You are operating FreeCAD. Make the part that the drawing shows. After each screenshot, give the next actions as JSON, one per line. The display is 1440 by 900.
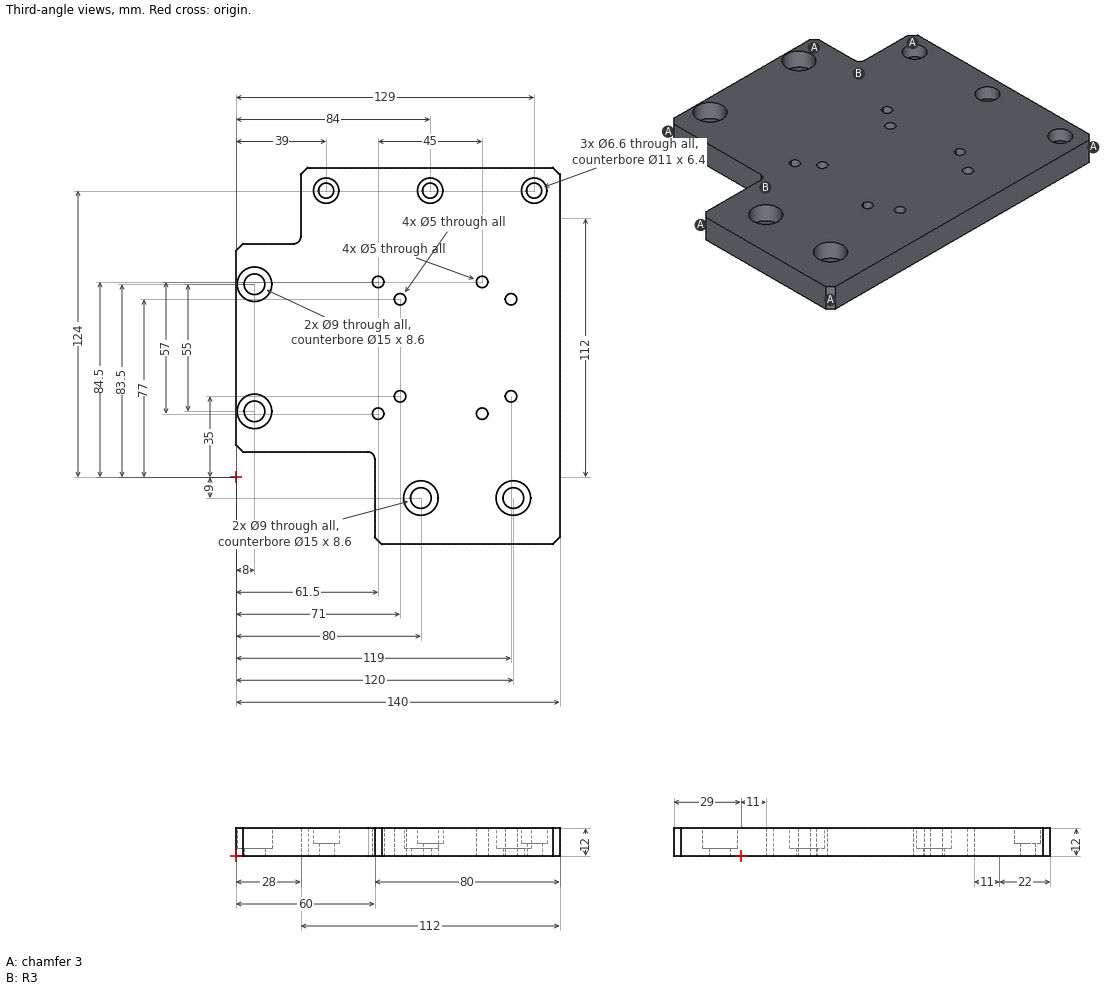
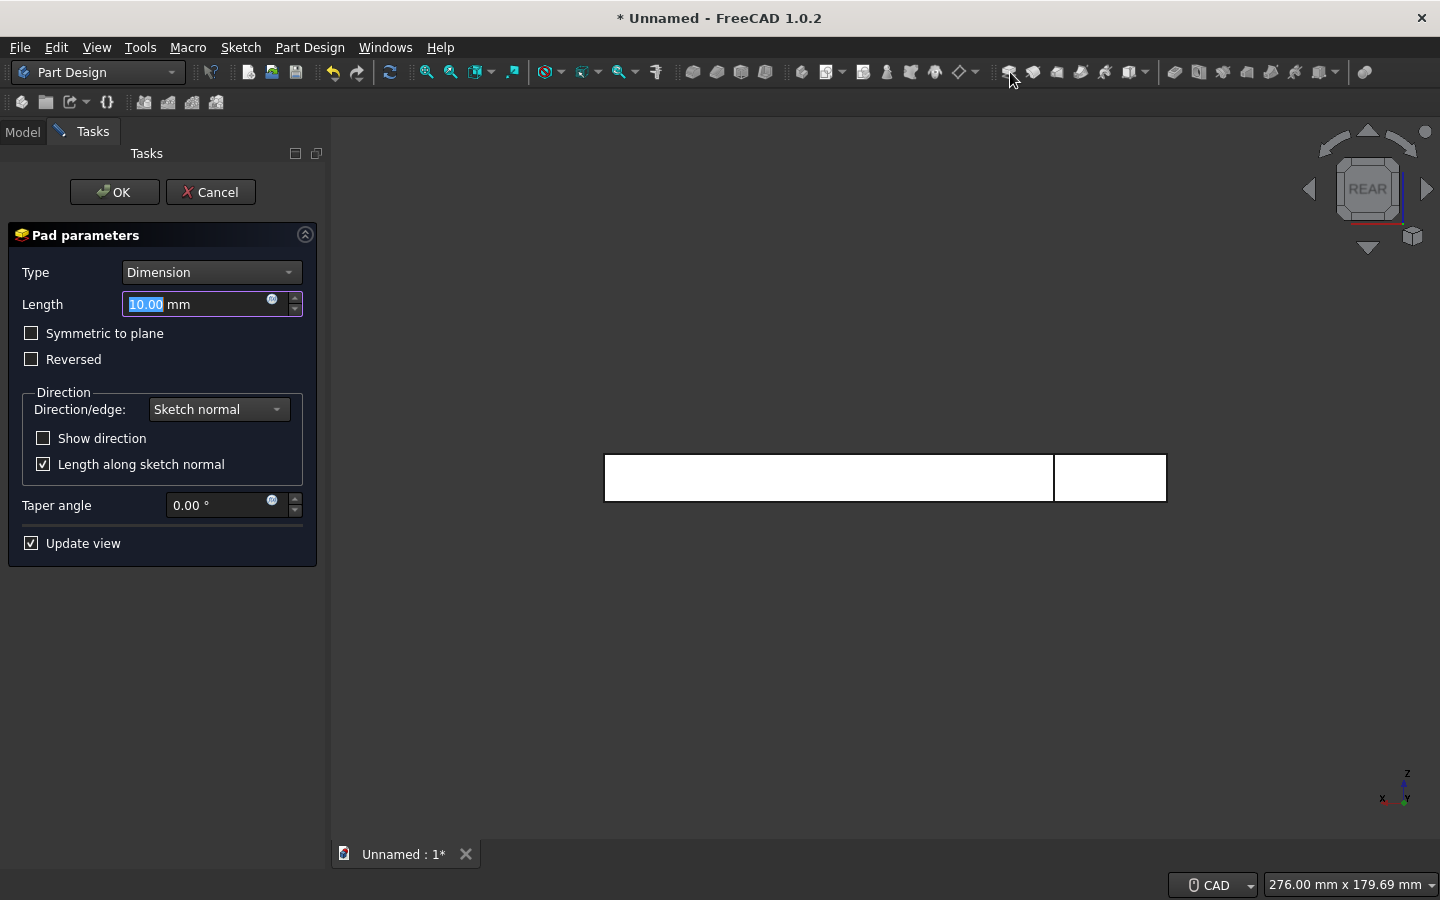
{"action": "type", "text": "22"}
{"action": "key", "text": "Tab"}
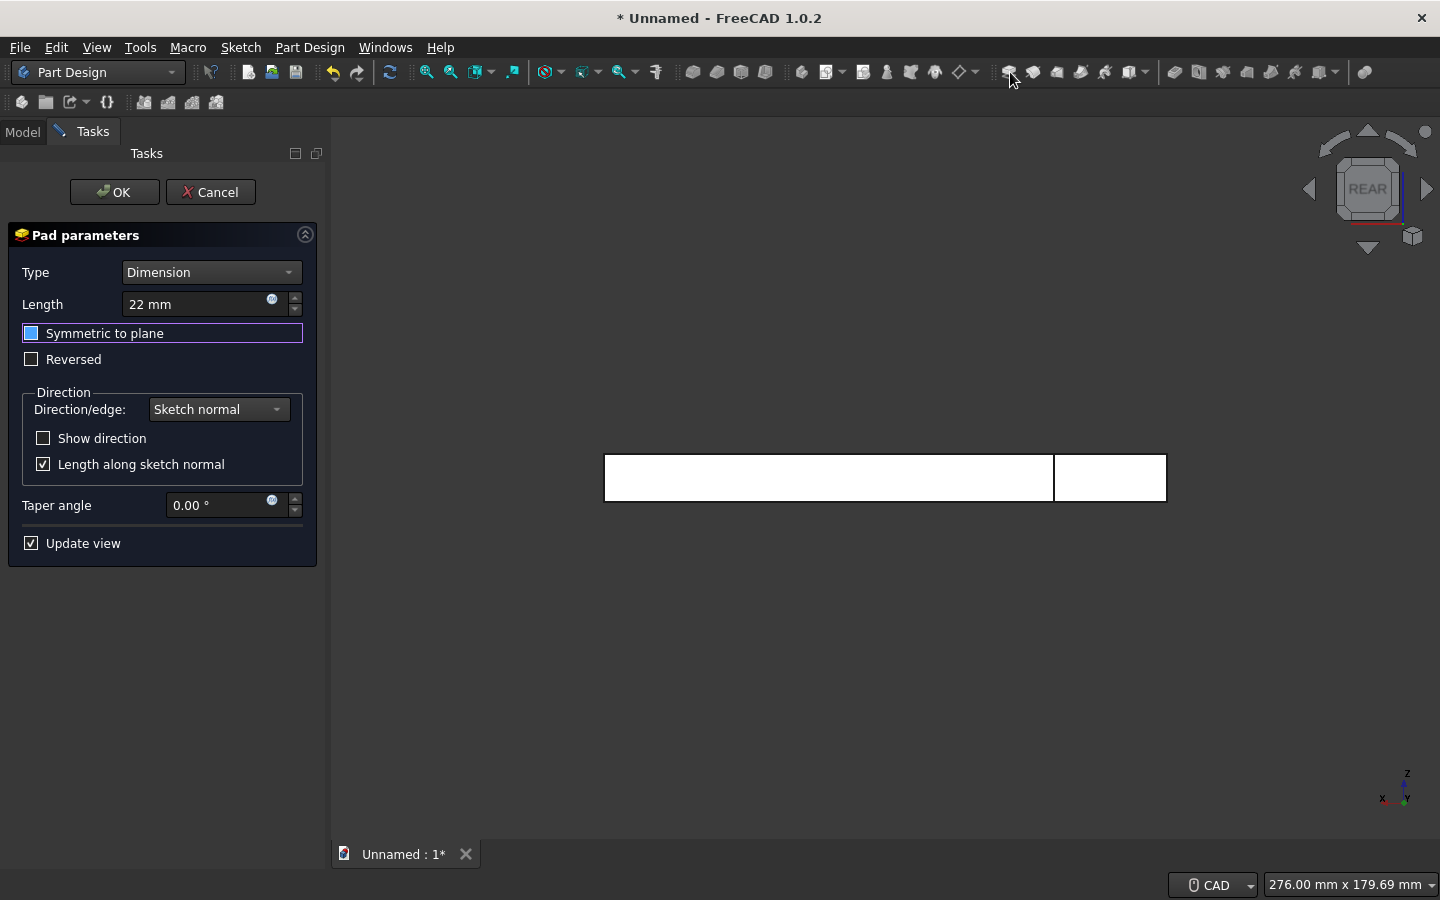
{"action": "left_click", "coordinate": [115, 192]}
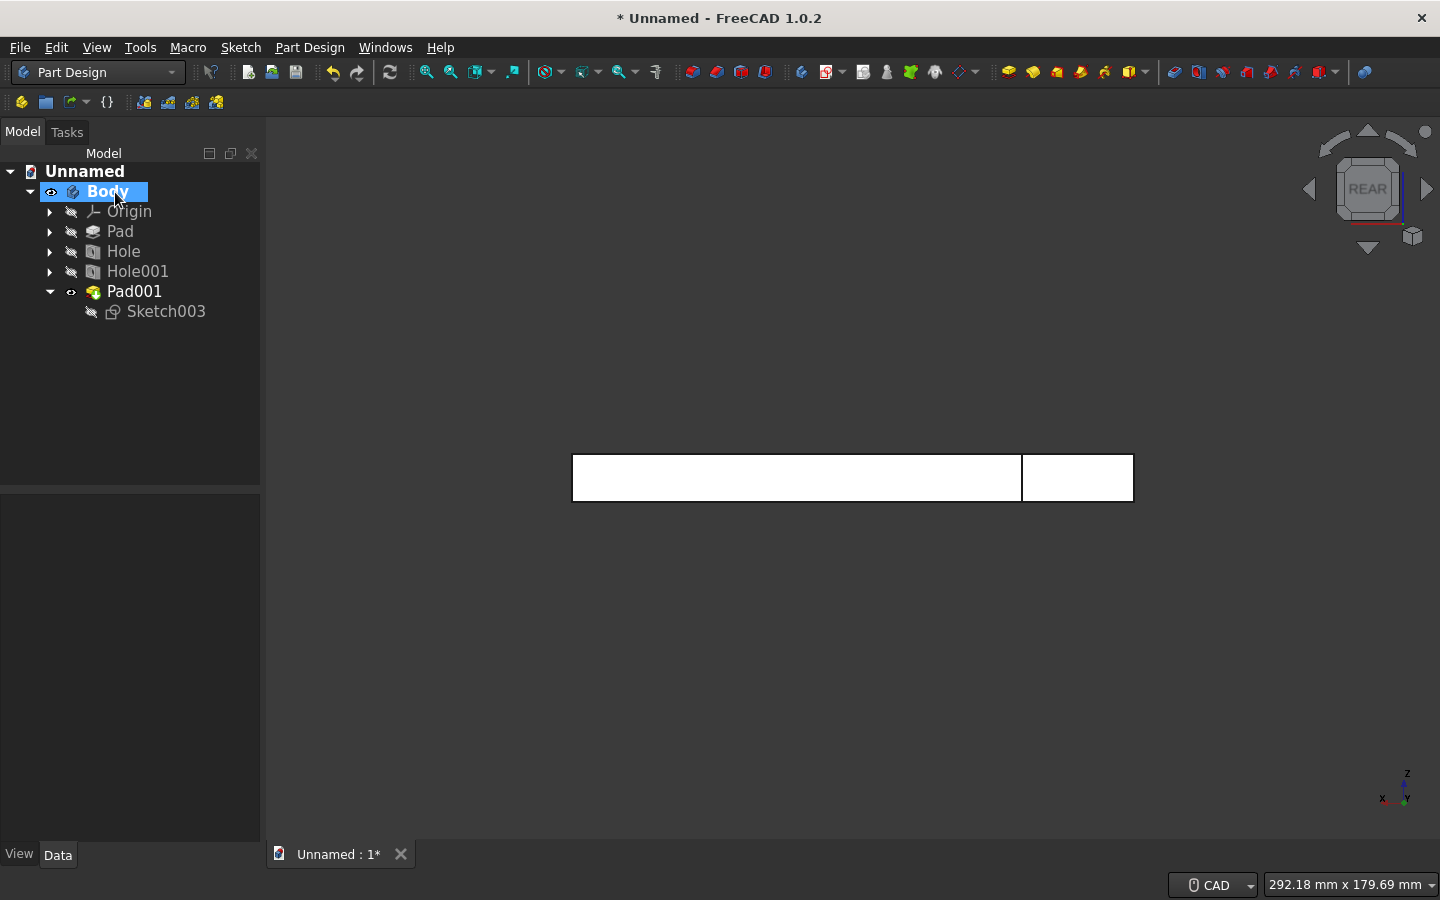
{"action": "left_click", "coordinate": [1046, 477]}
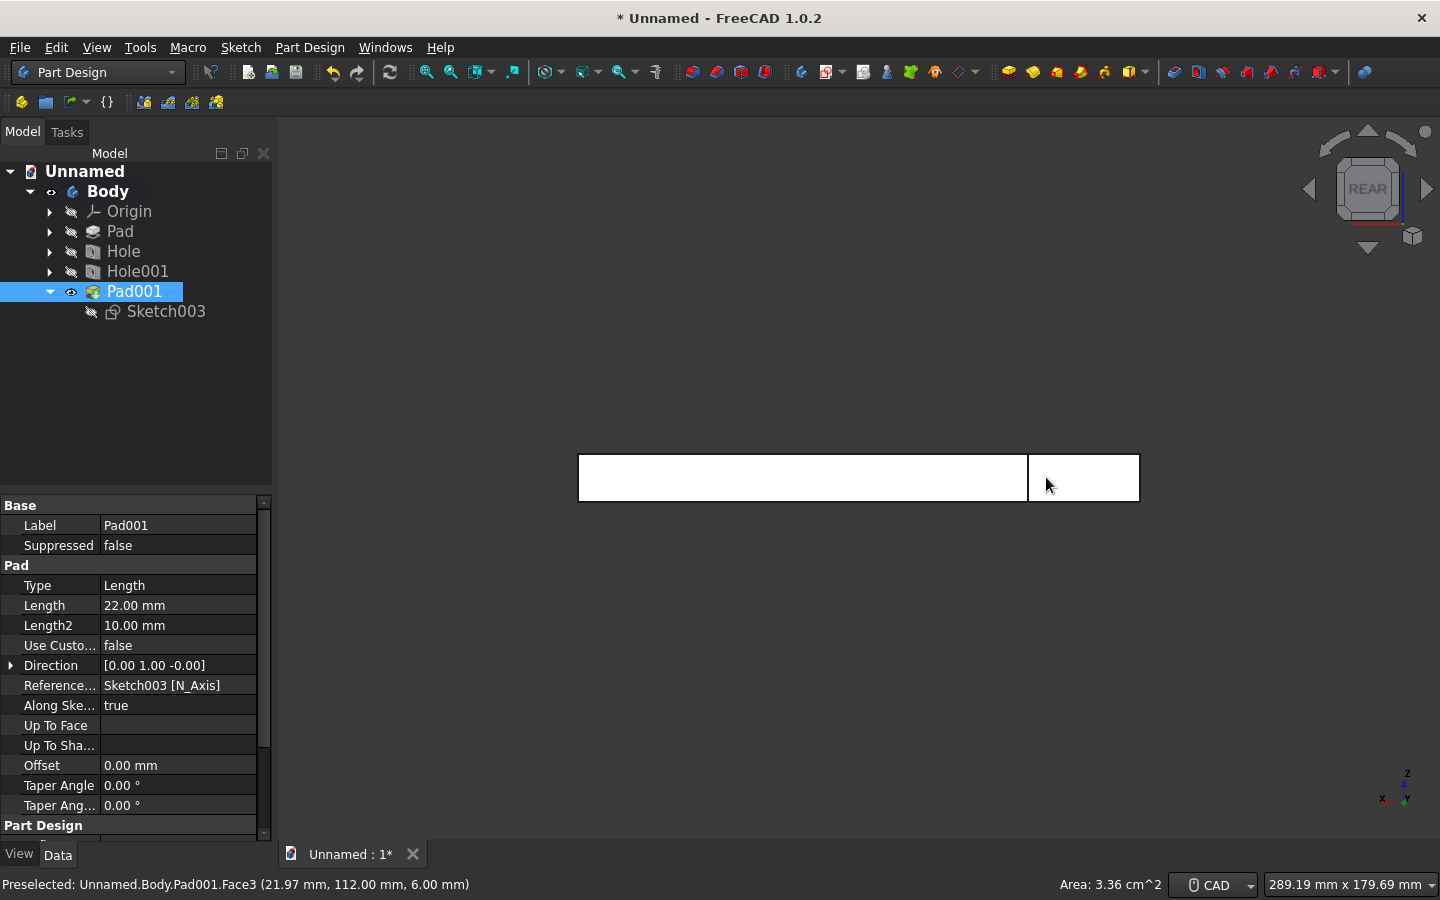
{"action": "left_click", "coordinate": [826, 72]}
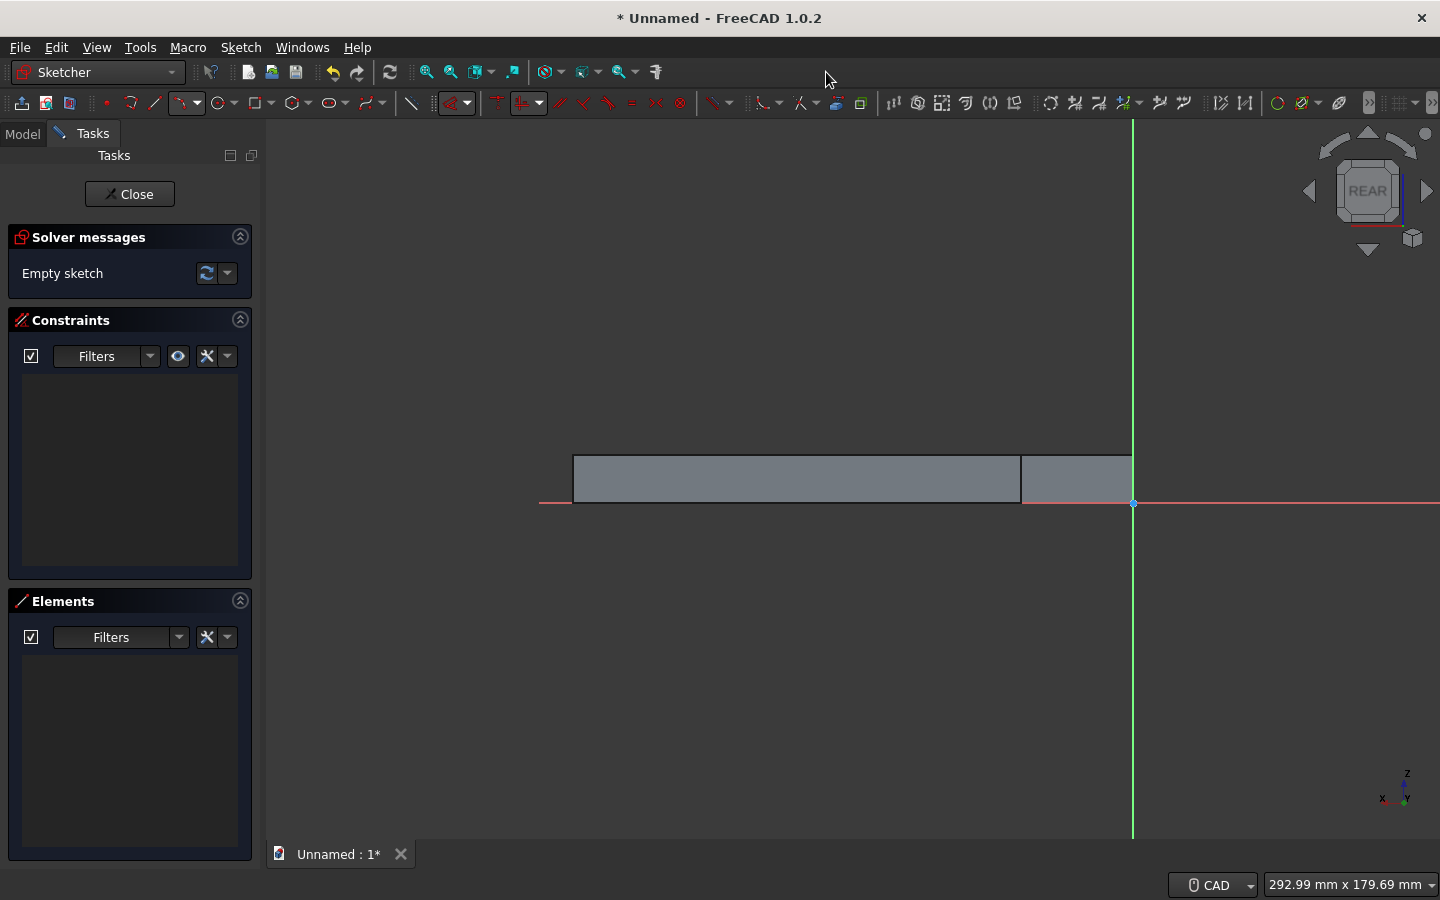
{"action": "left_click", "coordinate": [70, 104]}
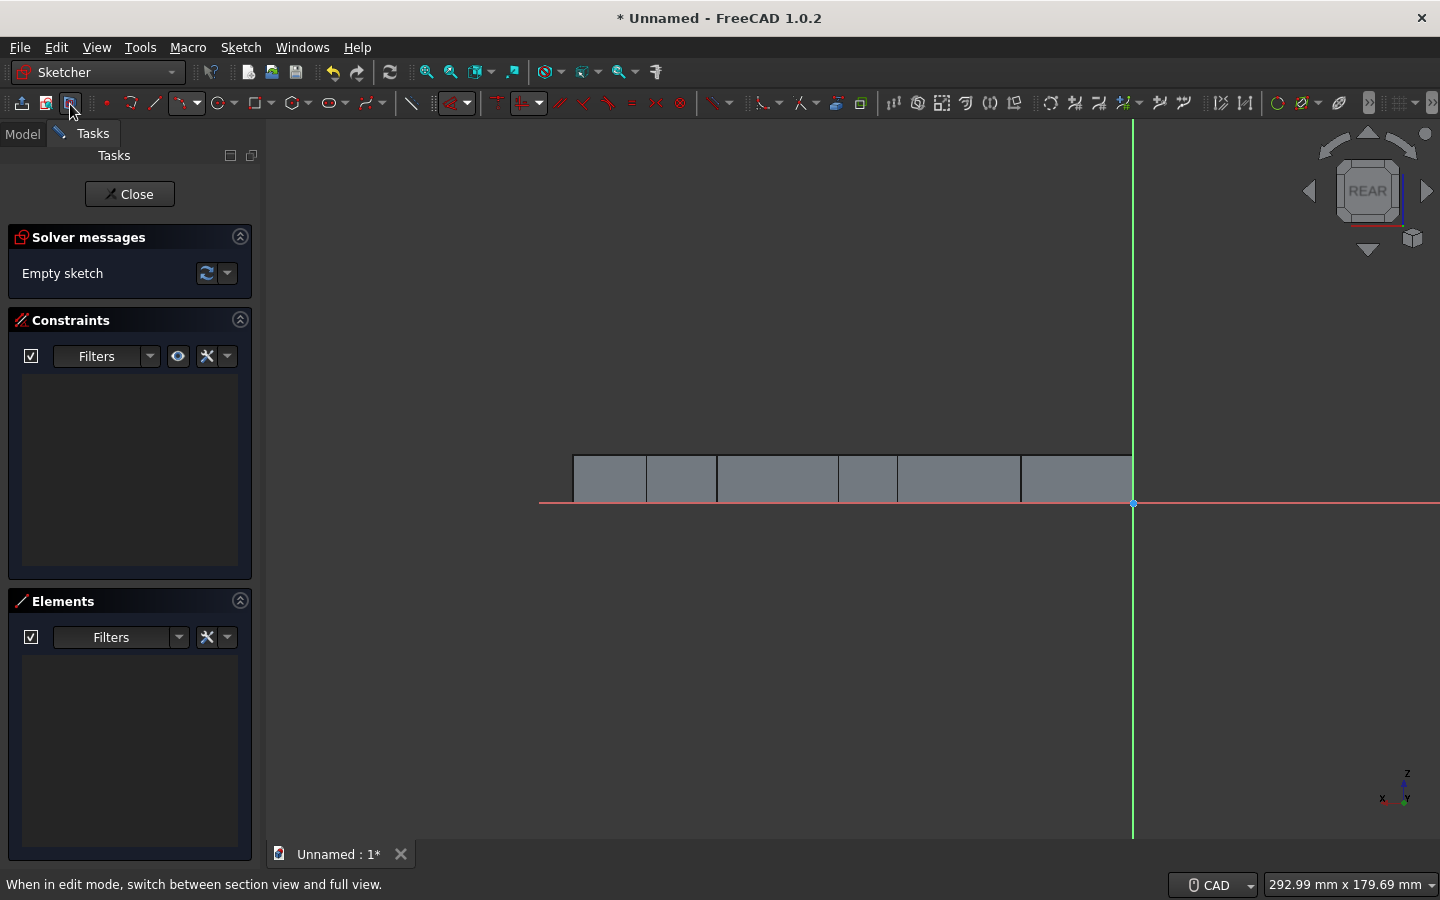
{"action": "scroll", "coordinate": [1135, 479], "scroll_direction": "up", "scroll_amount": 9}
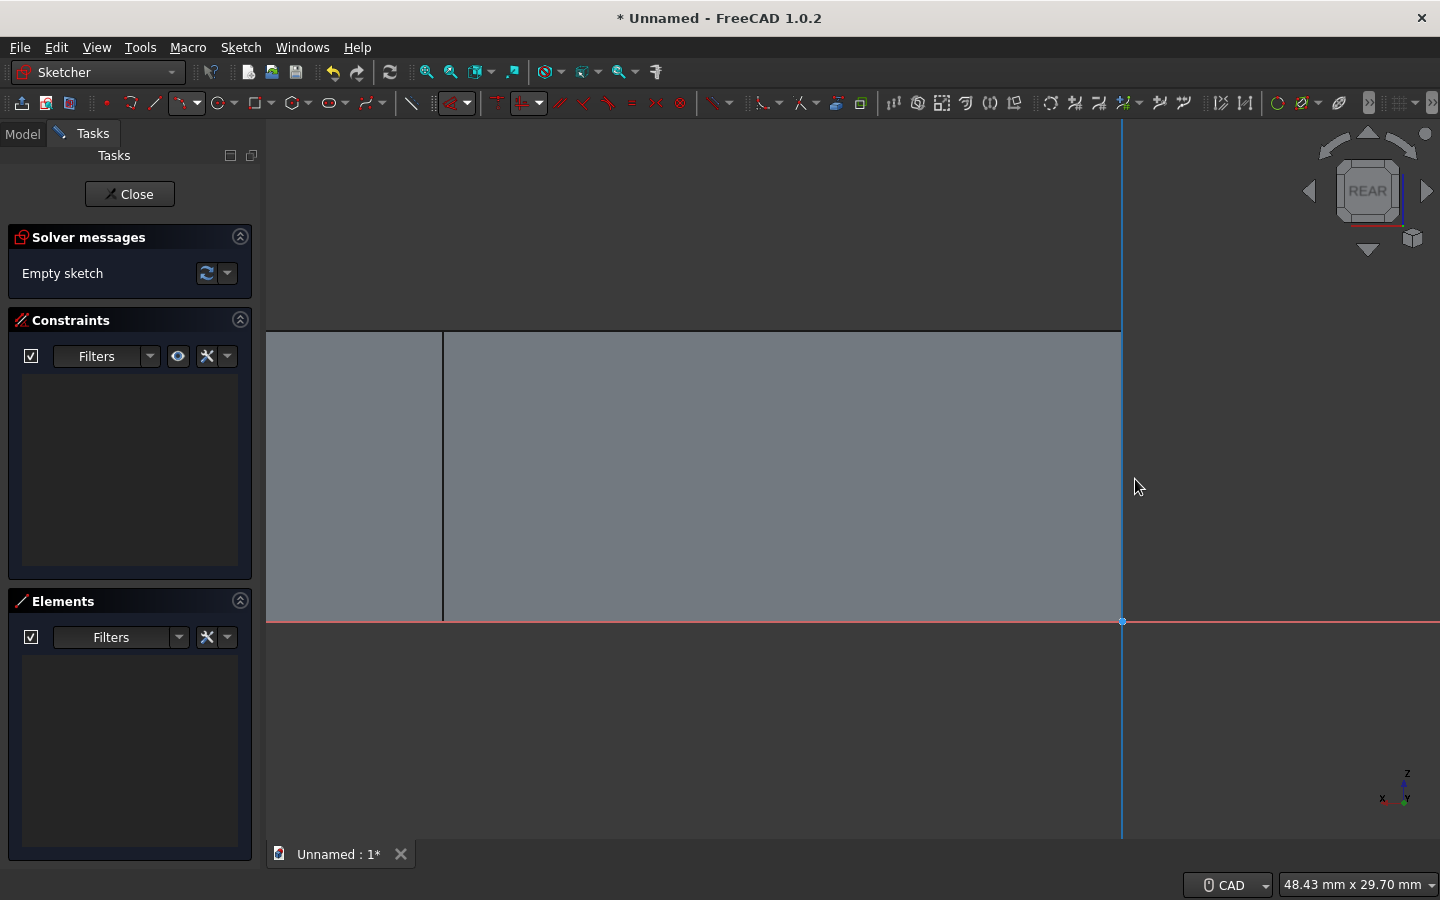
{"action": "left_click", "coordinate": [256, 104]}